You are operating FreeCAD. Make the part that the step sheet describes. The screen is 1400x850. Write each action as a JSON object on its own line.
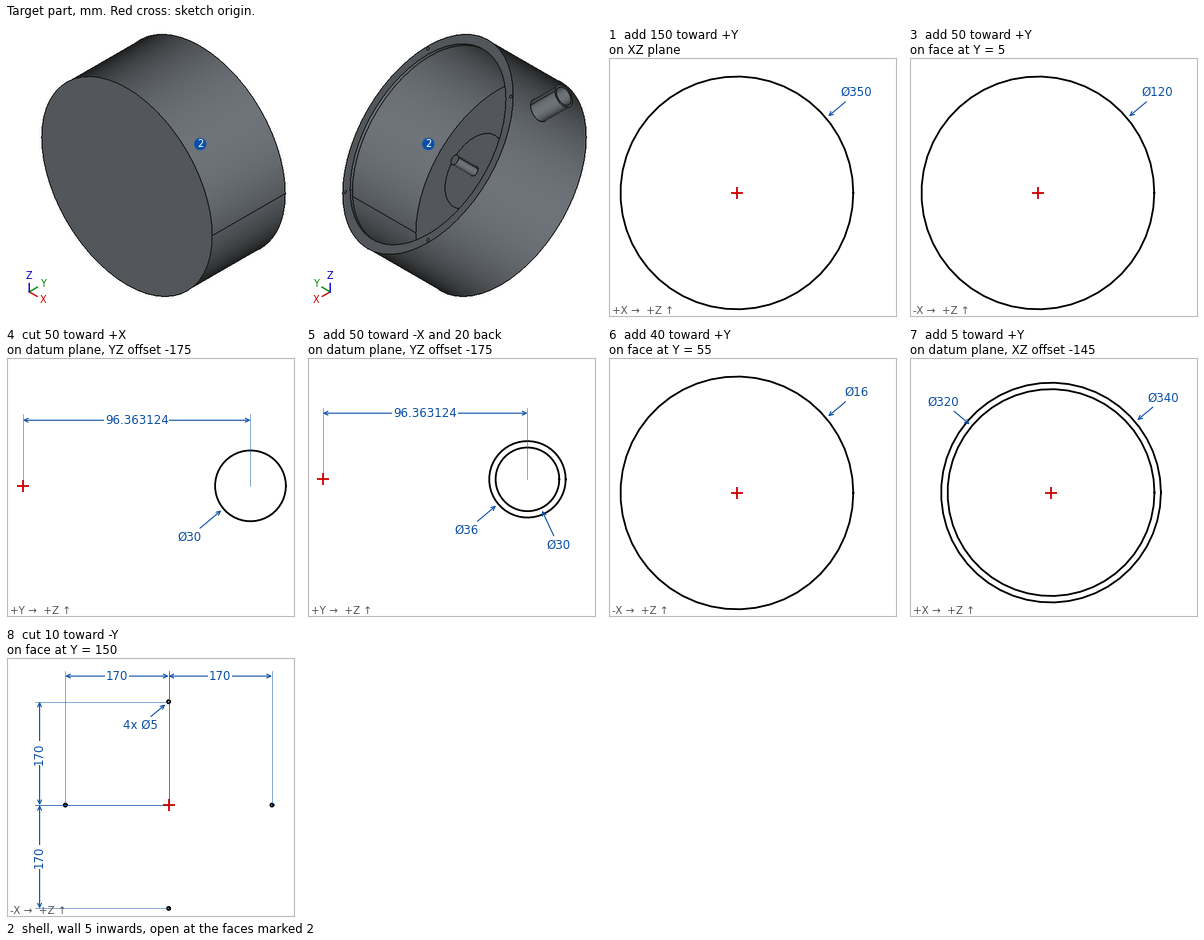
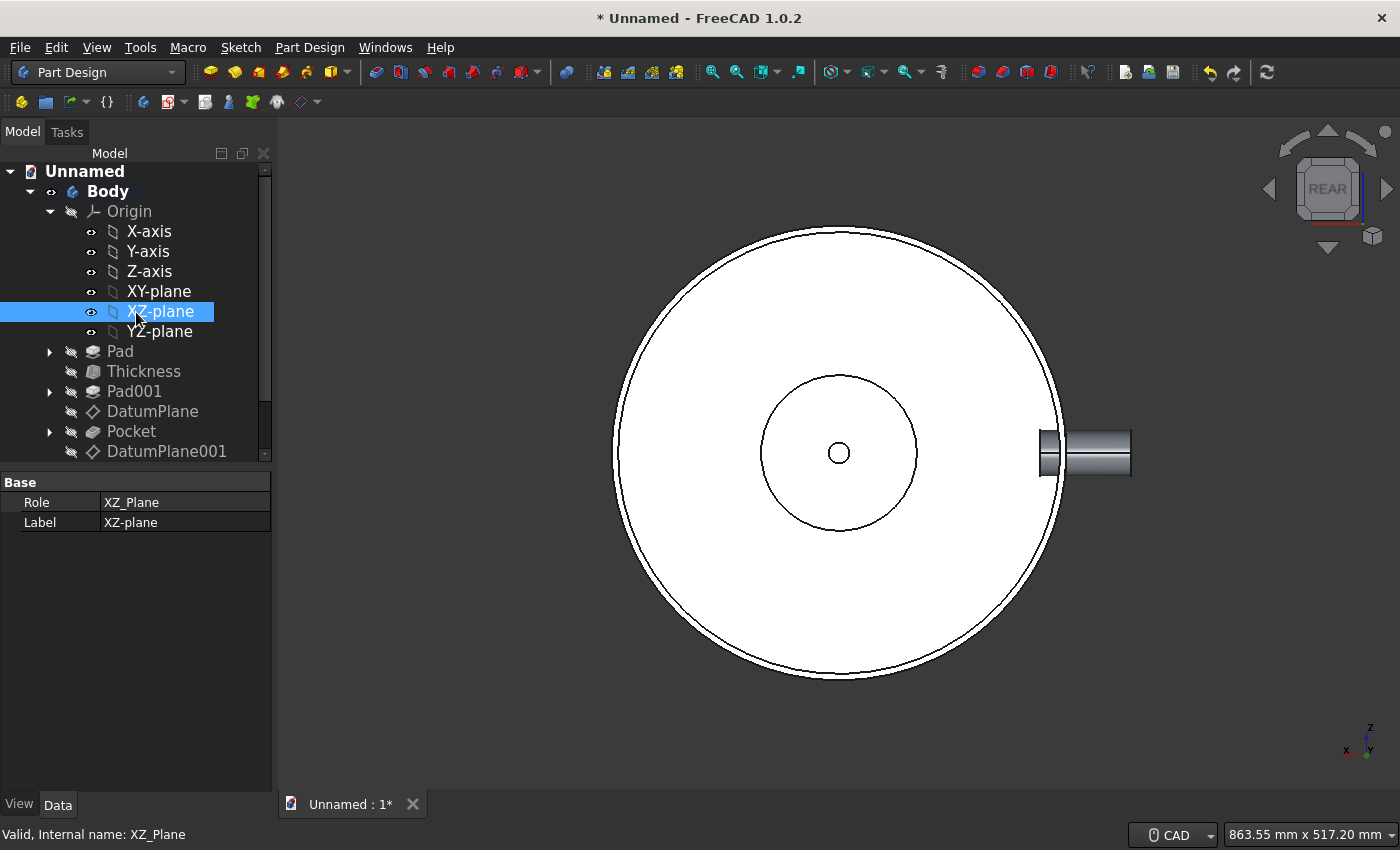
{"action": "left_click", "coordinate": [302, 102]}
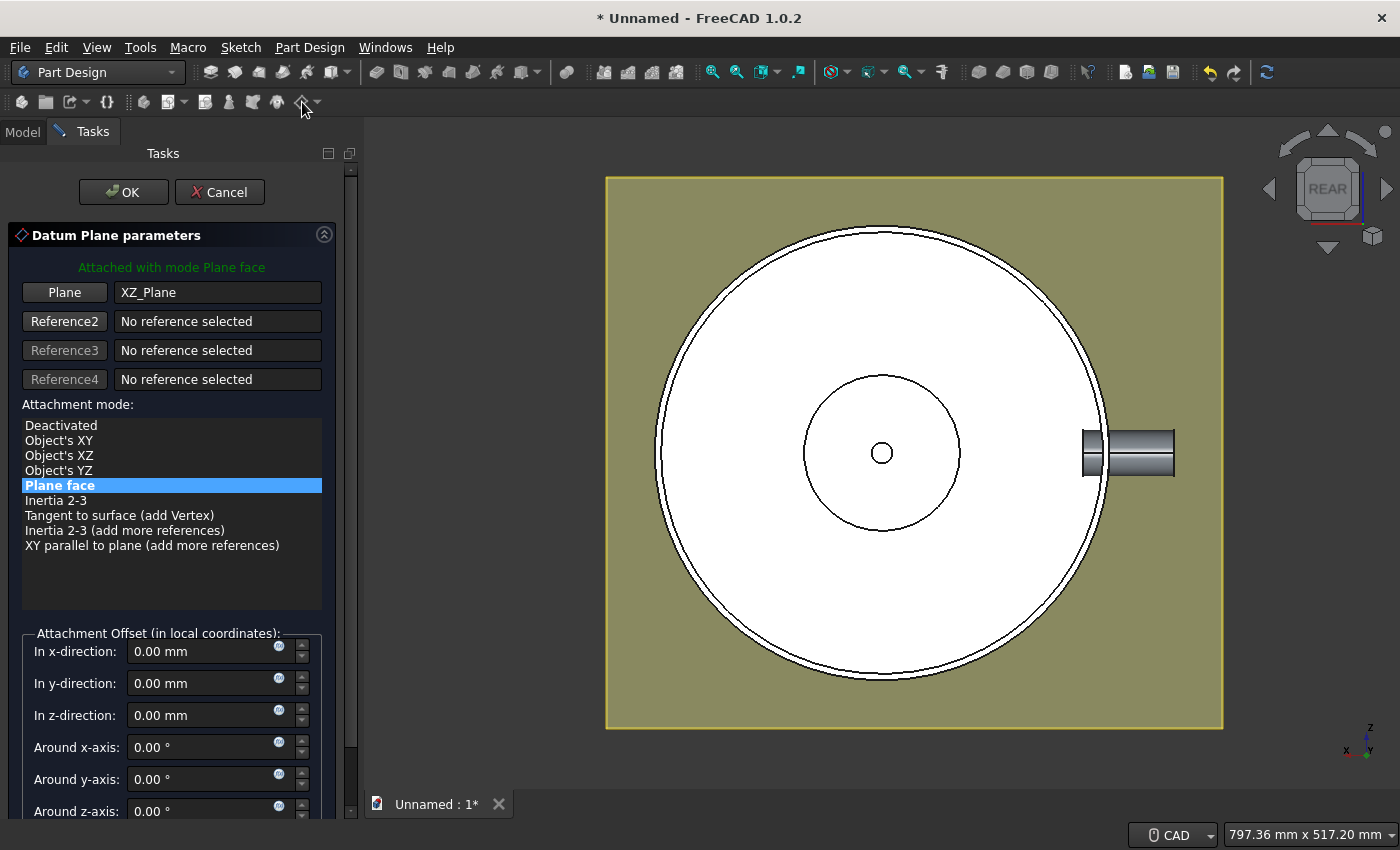
{"action": "triple_click", "coordinate": [210, 715]}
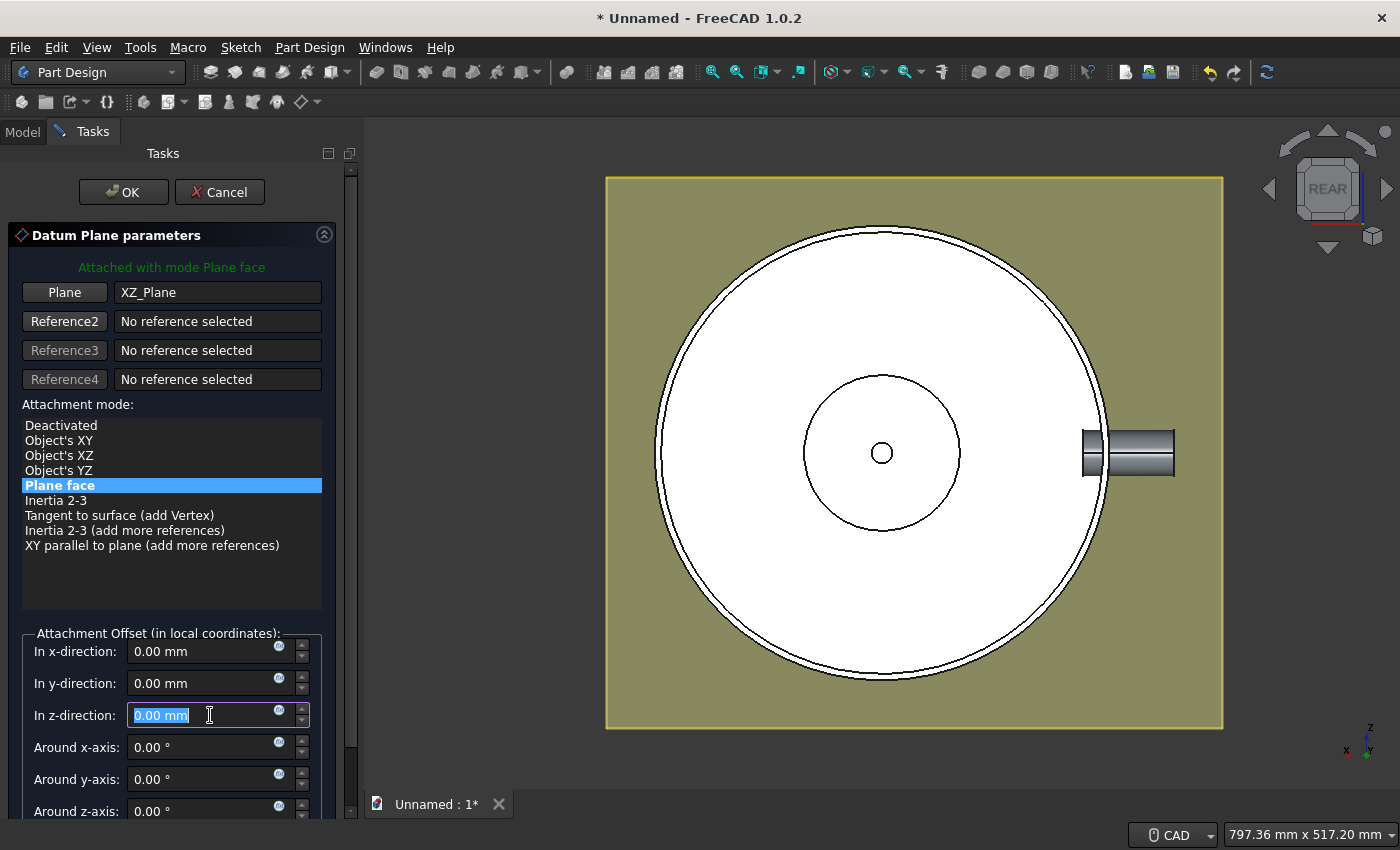
{"action": "type", "text": "-145"}
{"action": "key", "text": "Tab"}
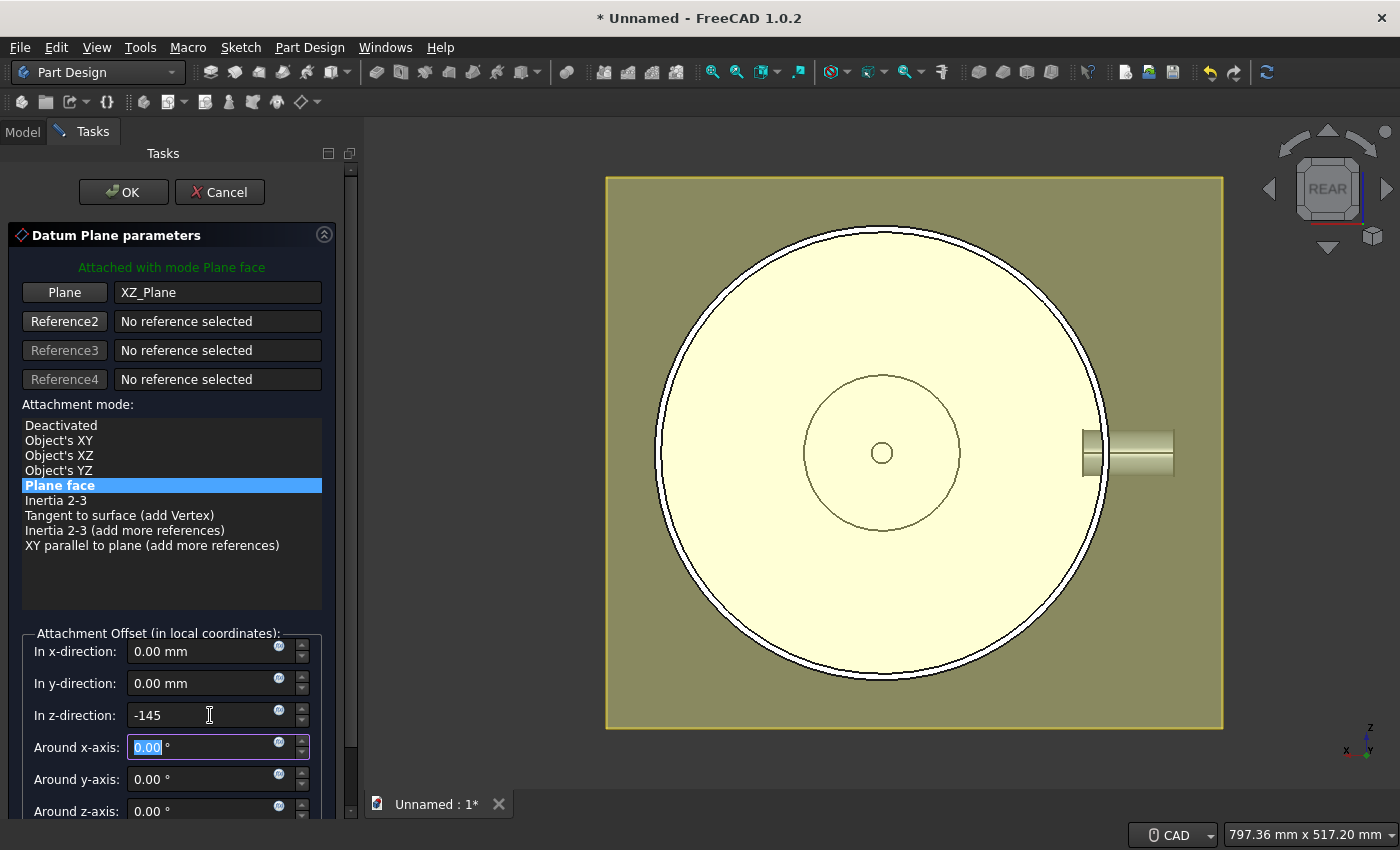
{"action": "left_click", "coordinate": [124, 192]}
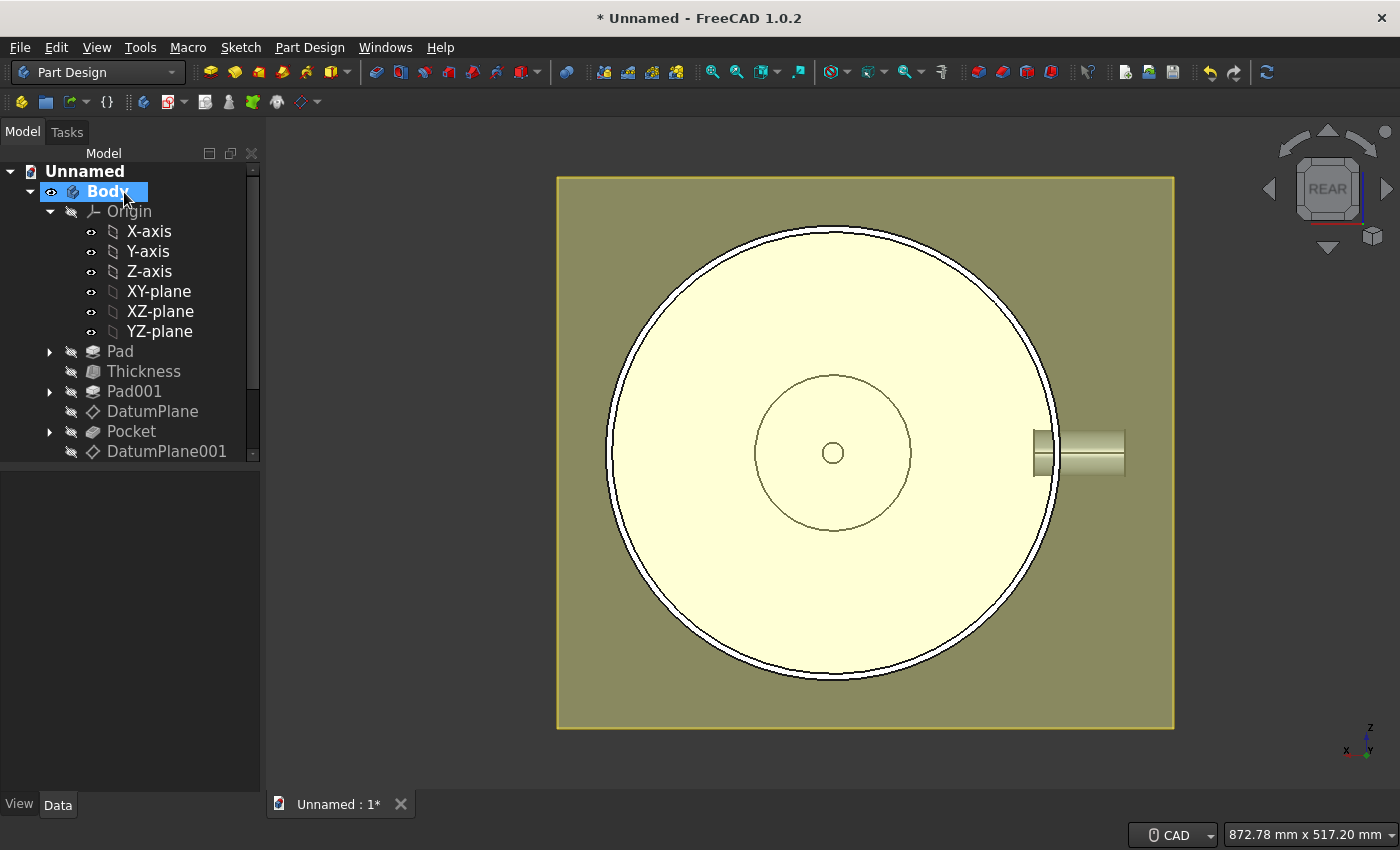
{"action": "scroll", "coordinate": [100, 307], "scroll_direction": "down", "scroll_amount": 3}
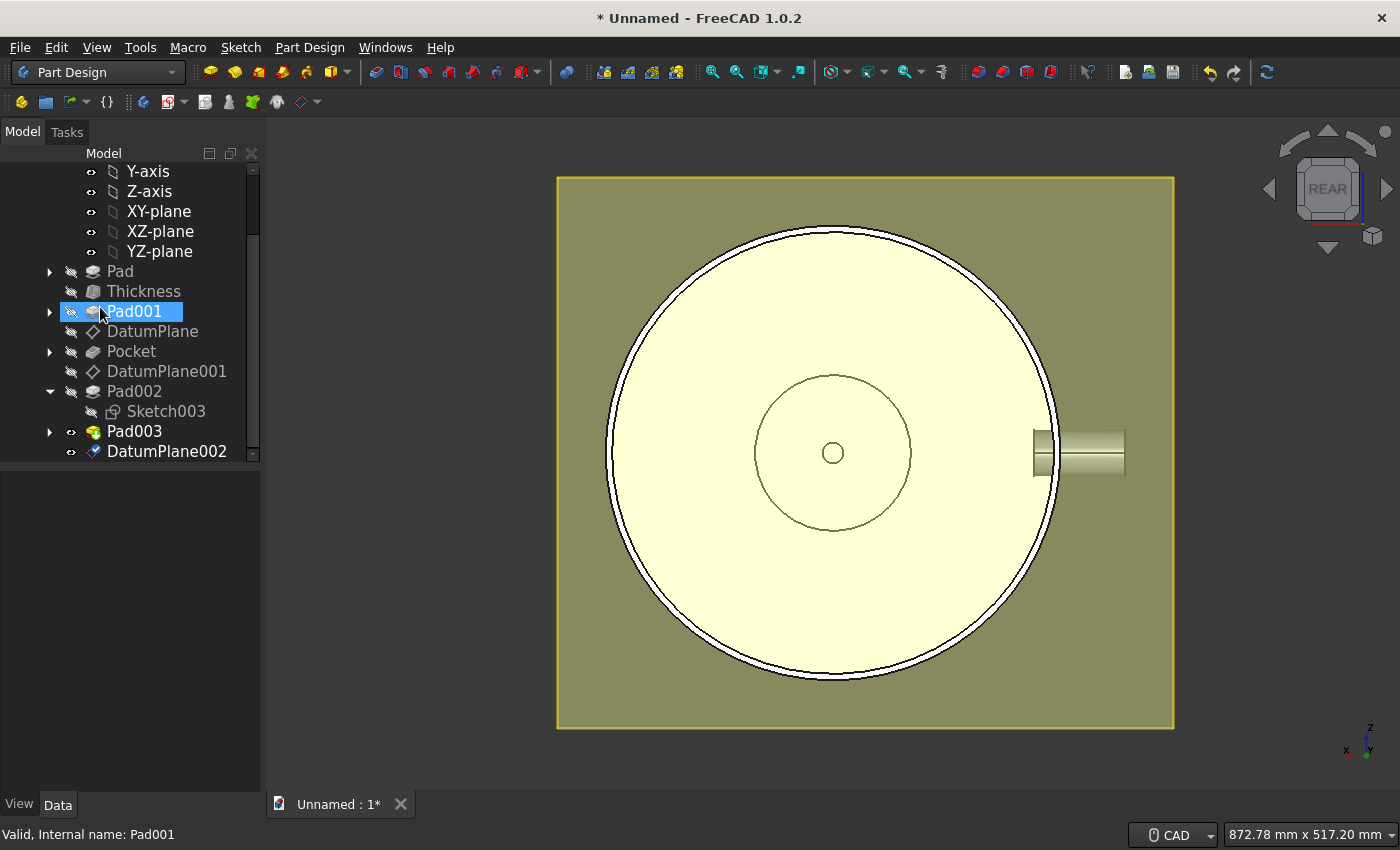
{"action": "left_click", "coordinate": [116, 452]}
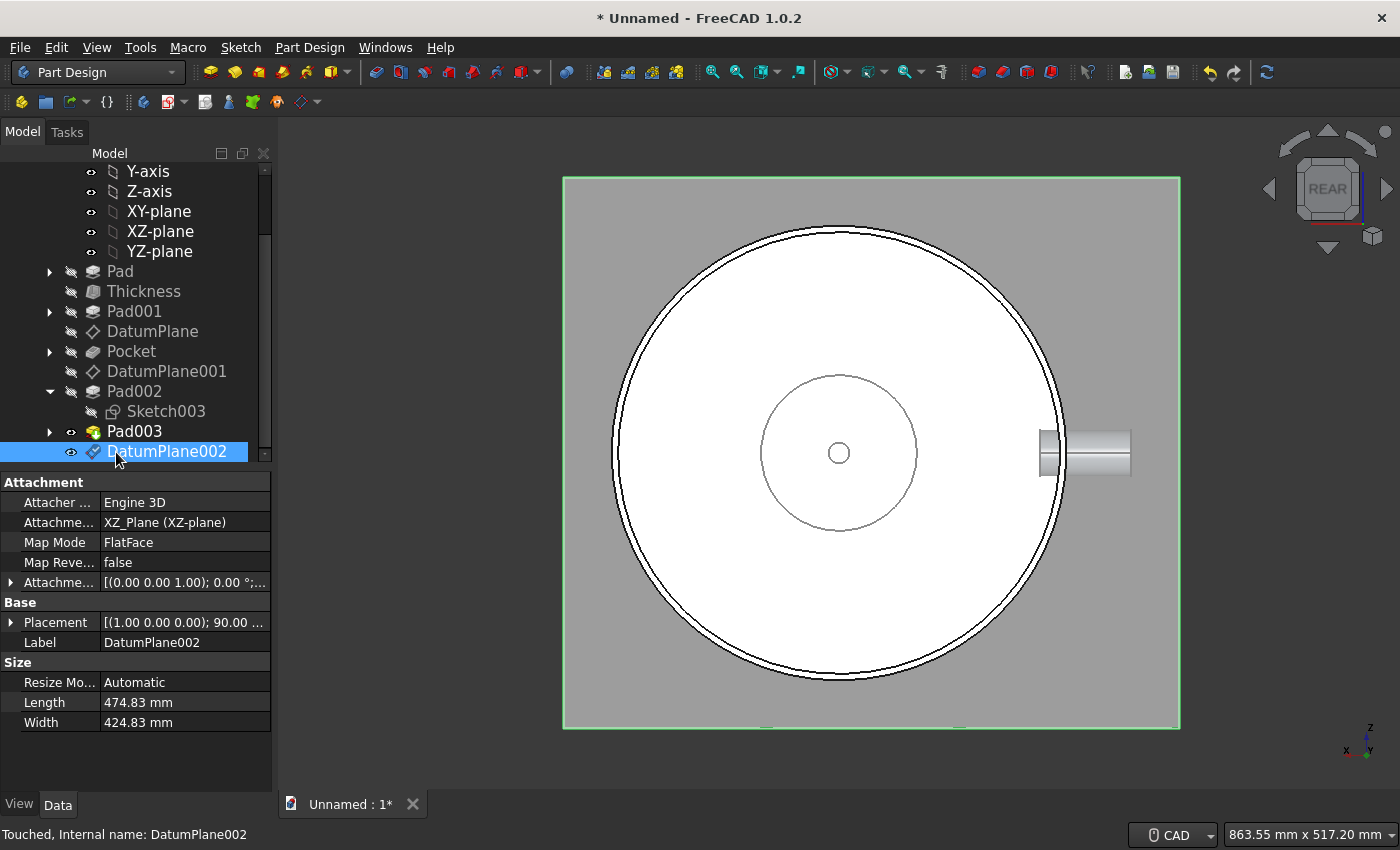
{"action": "left_click", "coordinate": [168, 102]}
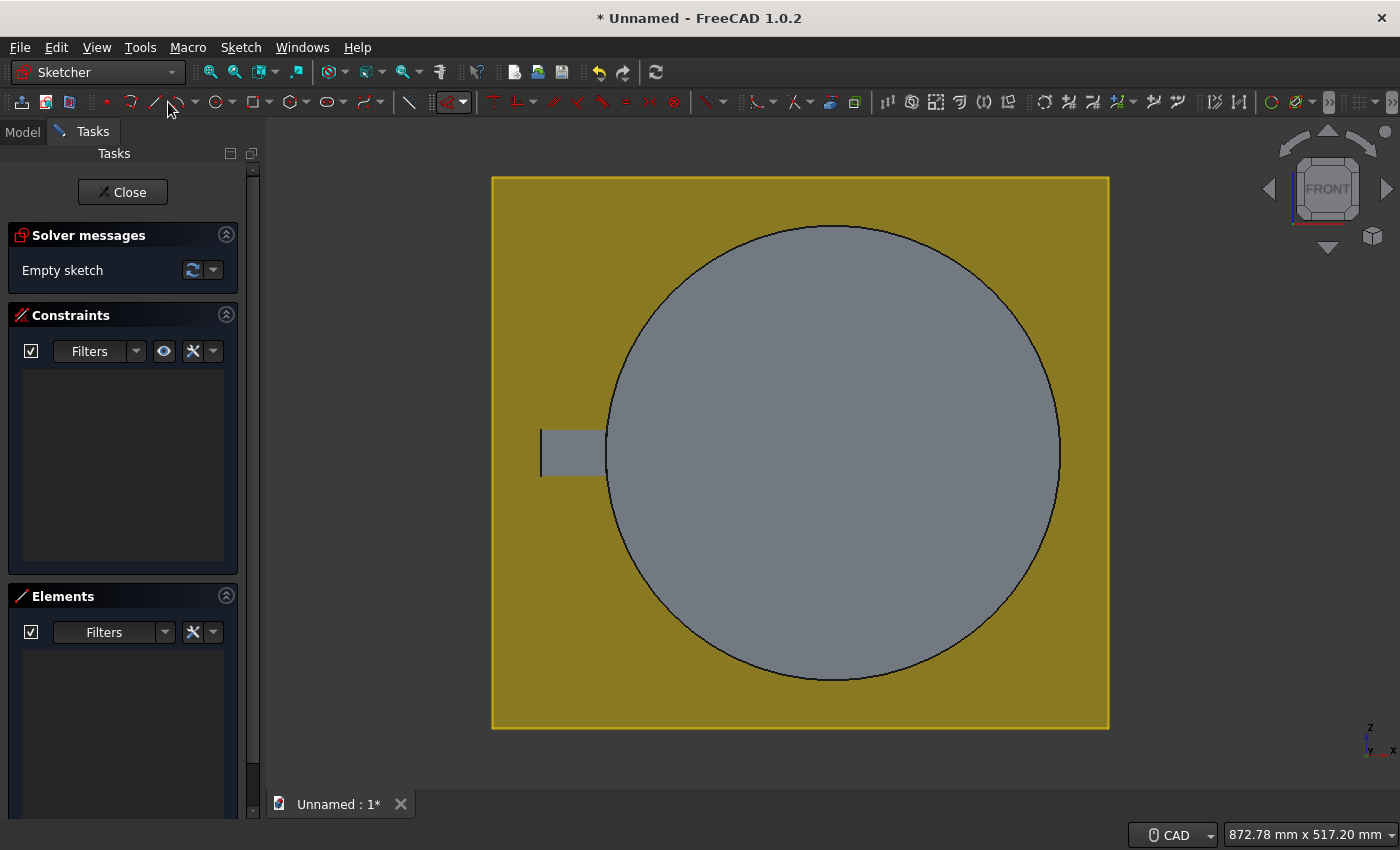
{"action": "left_click", "coordinate": [70, 102]}